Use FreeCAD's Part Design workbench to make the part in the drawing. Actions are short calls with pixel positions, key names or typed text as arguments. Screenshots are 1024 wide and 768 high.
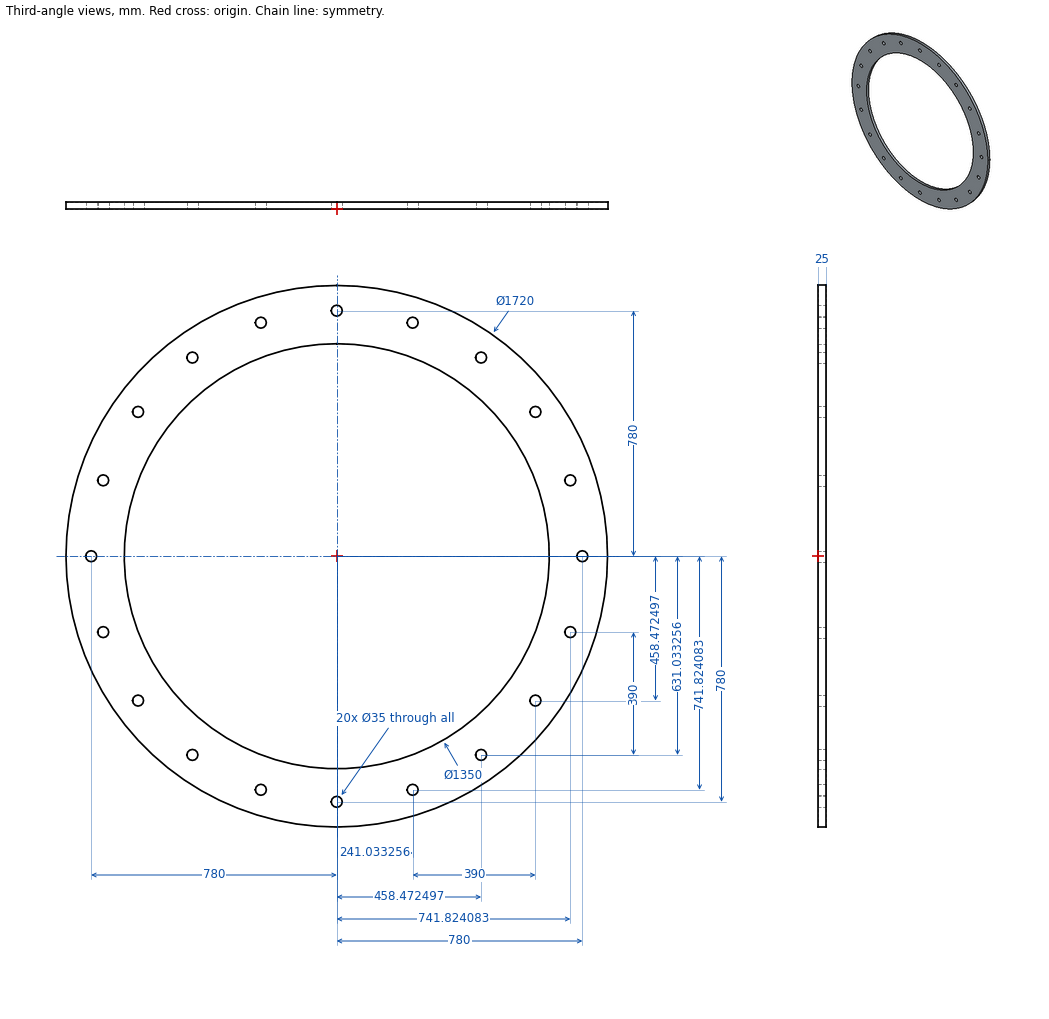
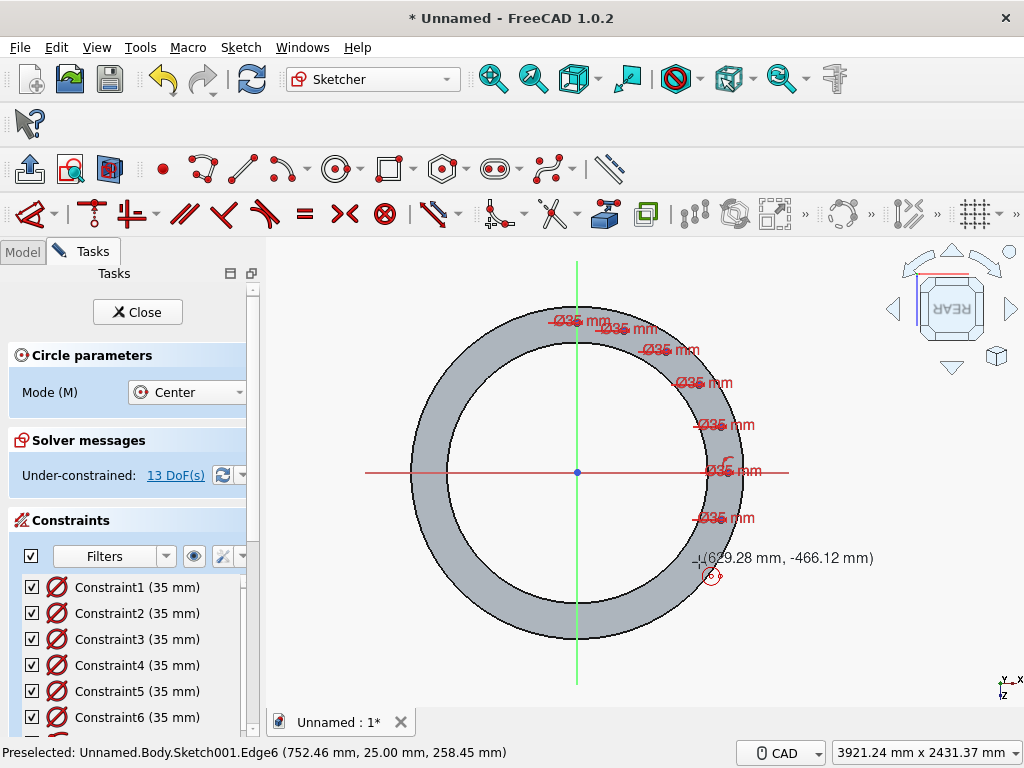
click(699, 562)
move(702, 559)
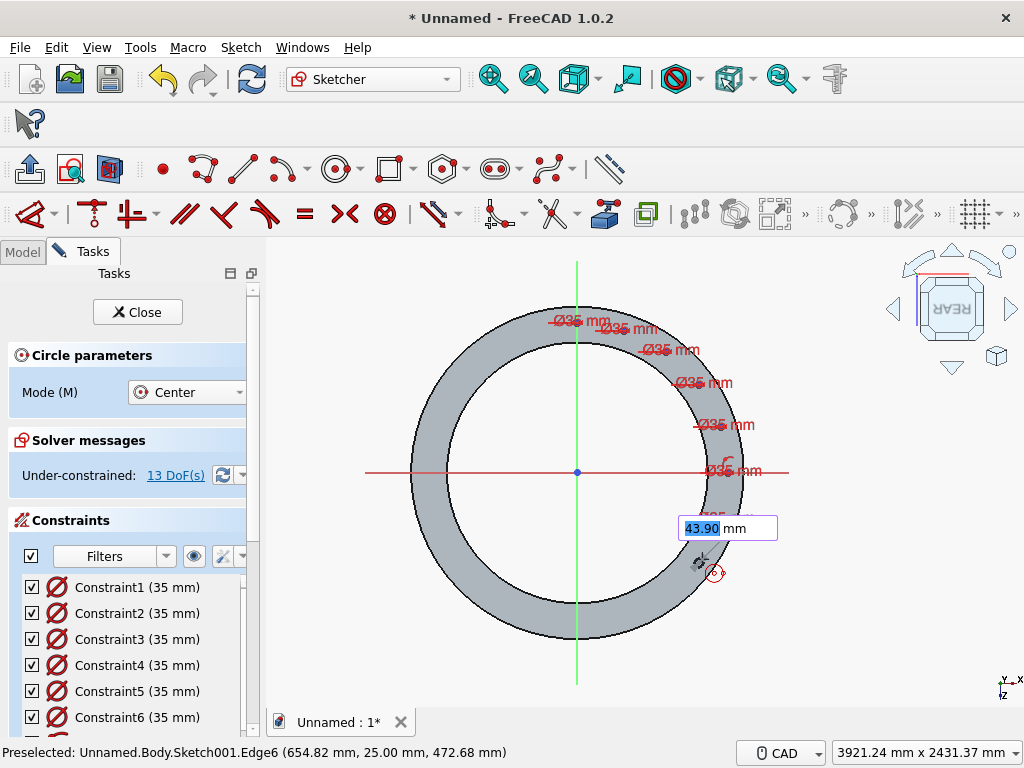
text(35)
key(Return)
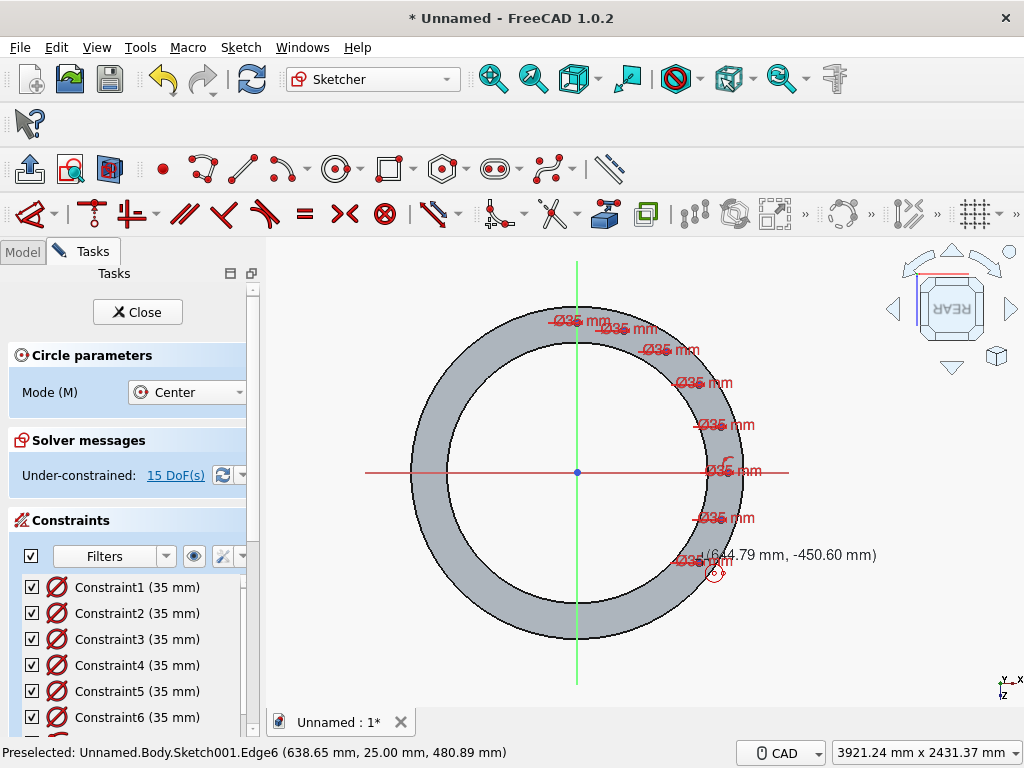
scroll(666, 595, up, 10)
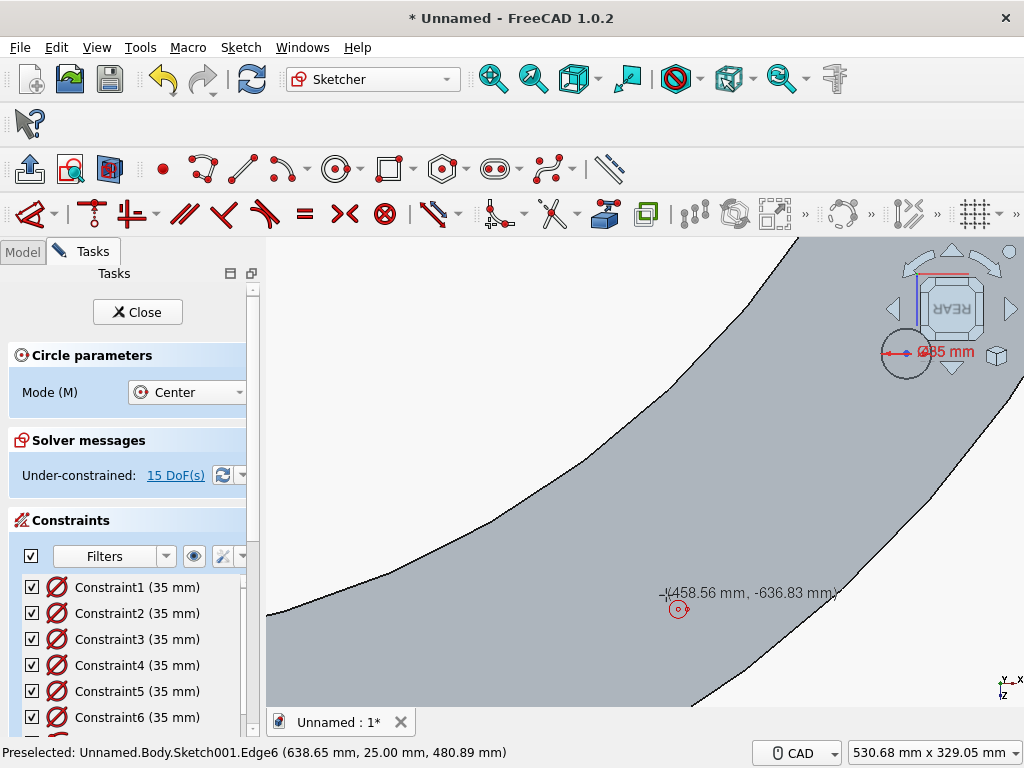
scroll(666, 595, down, 10)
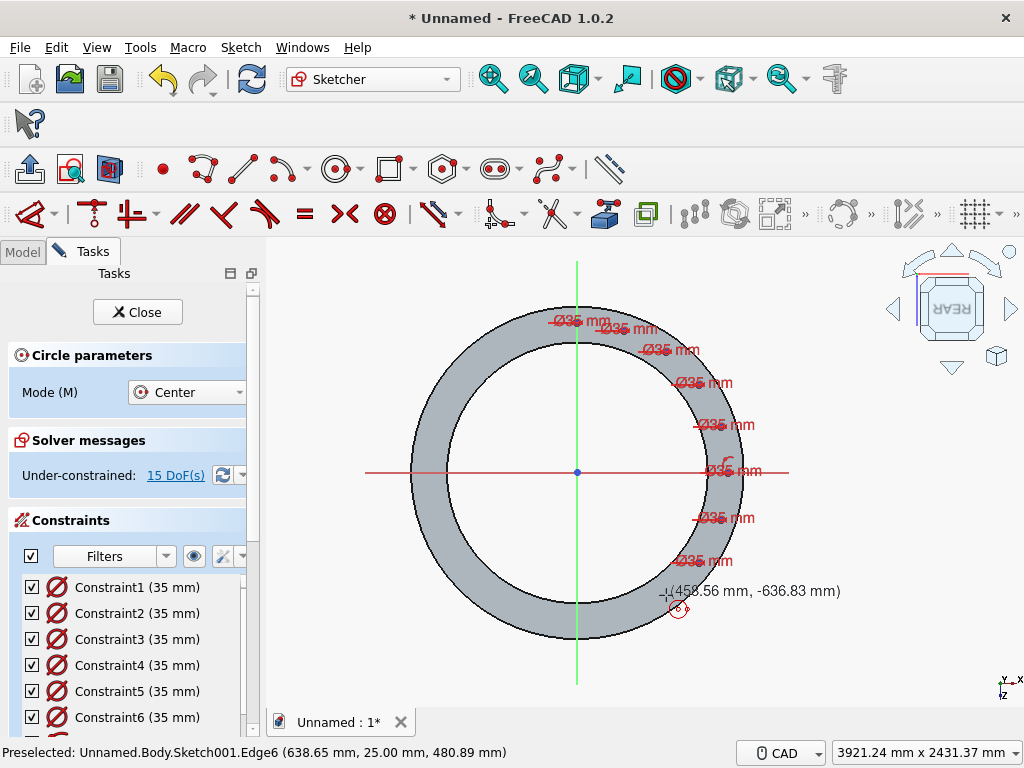
click(666, 595)
move(668, 592)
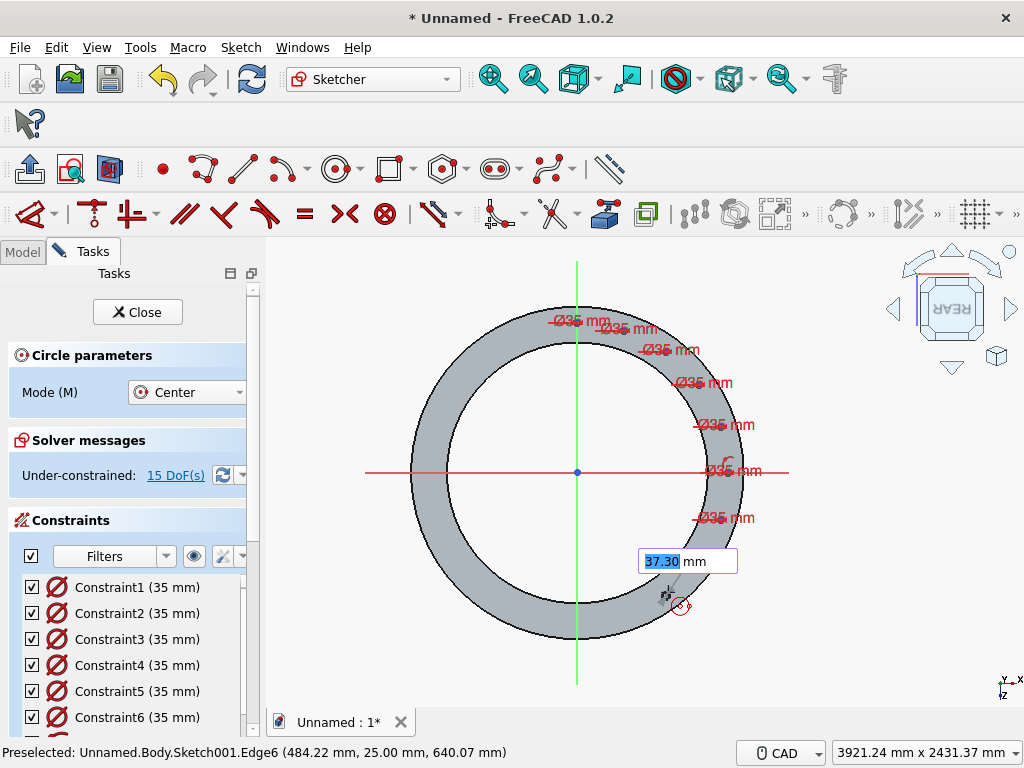
text(35)
key(Return)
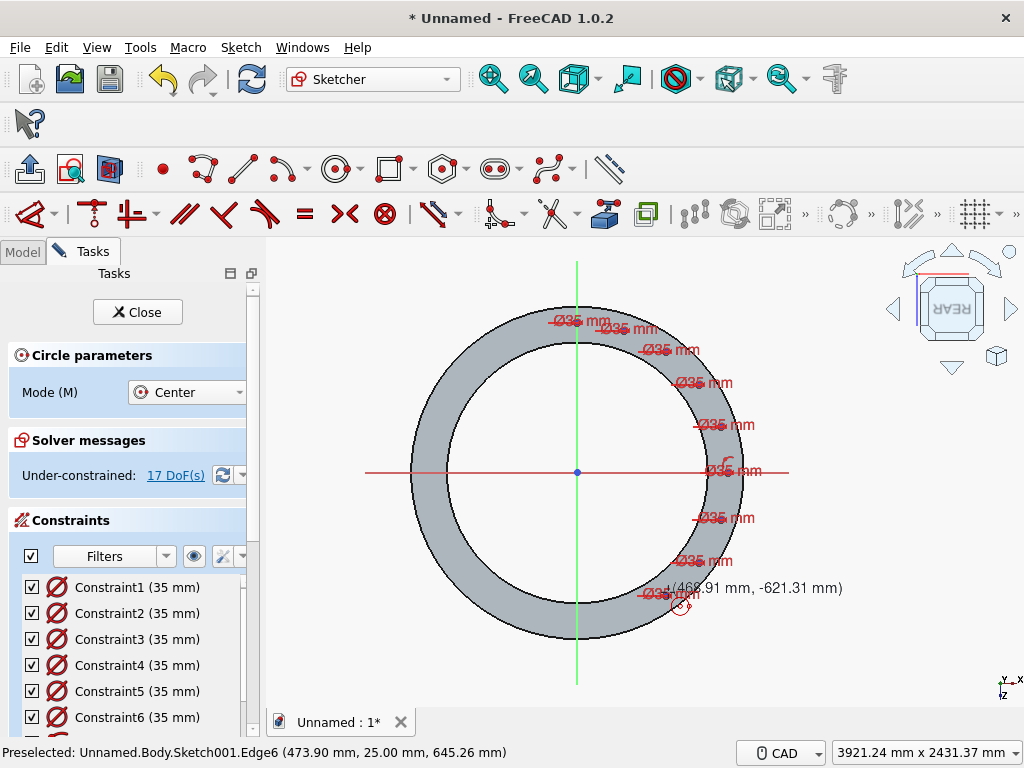
scroll(624, 616, up, 10)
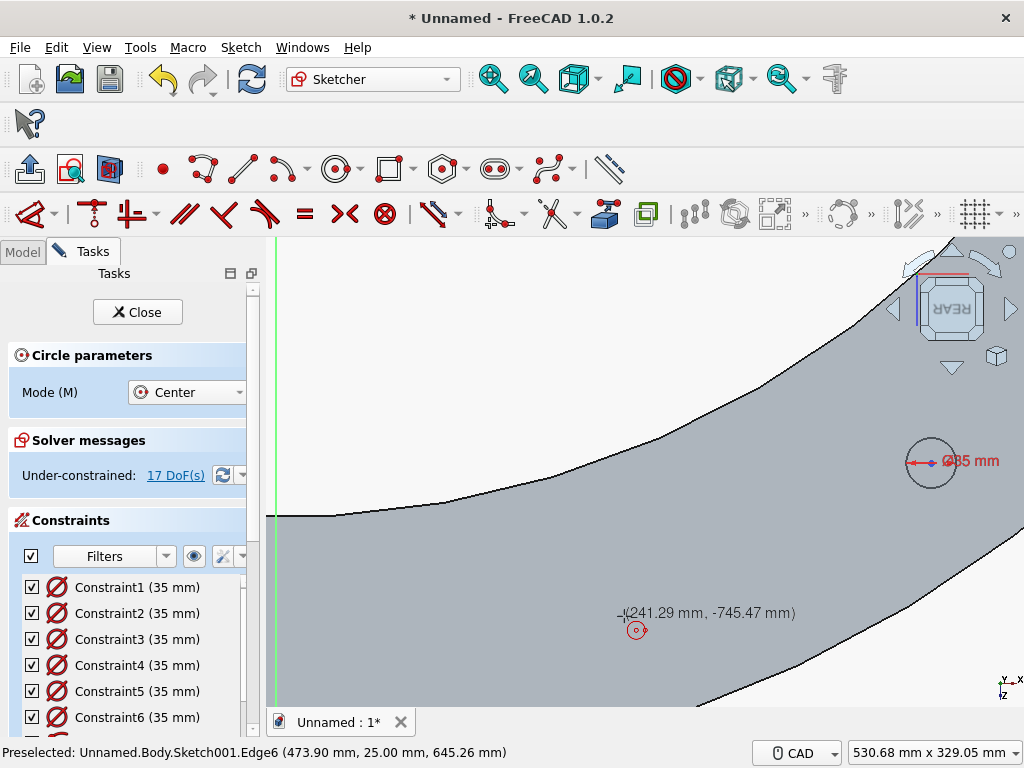
scroll(623, 616, down, 10)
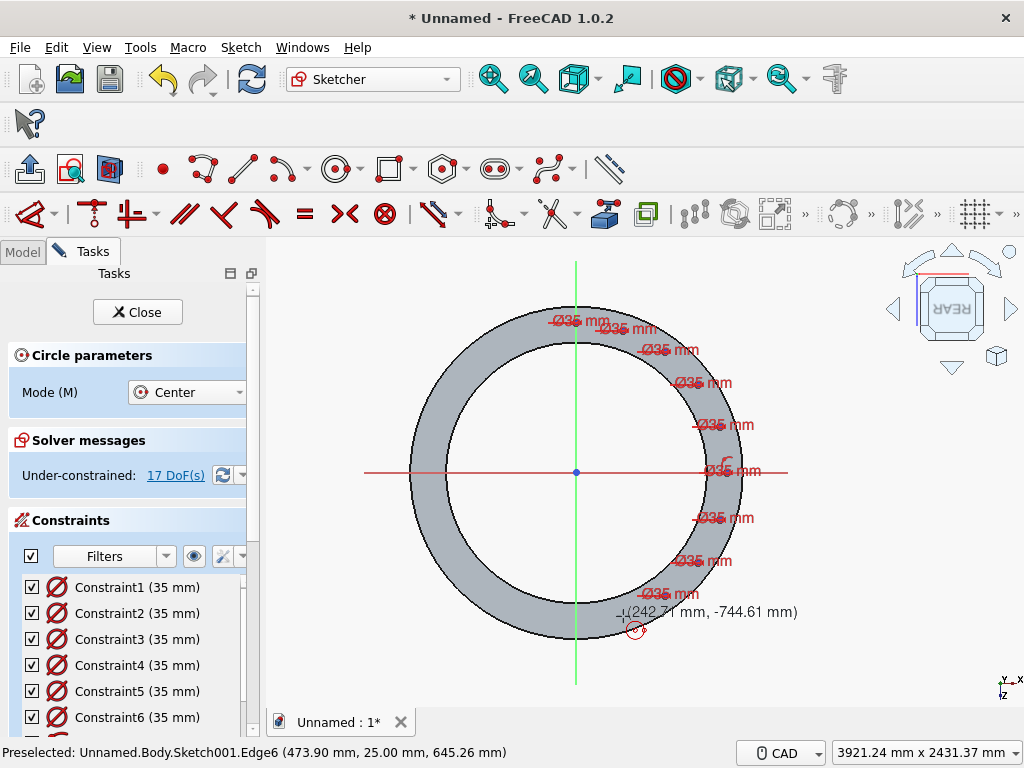
click(623, 616)
move(625, 614)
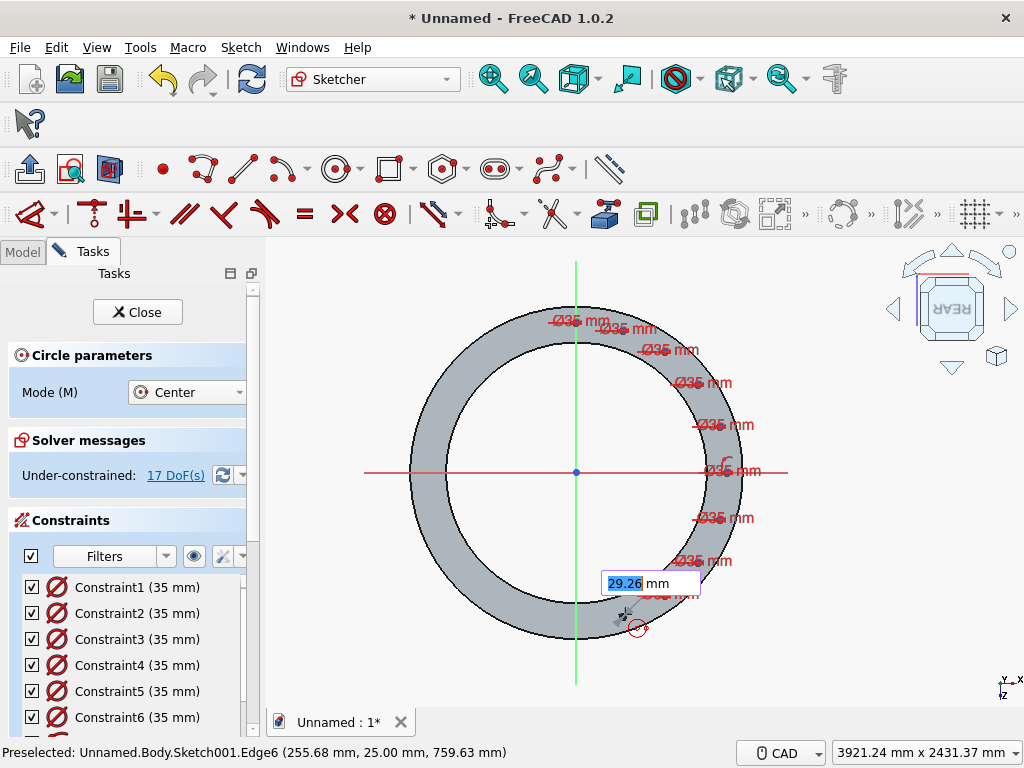
text(35)
key(Return)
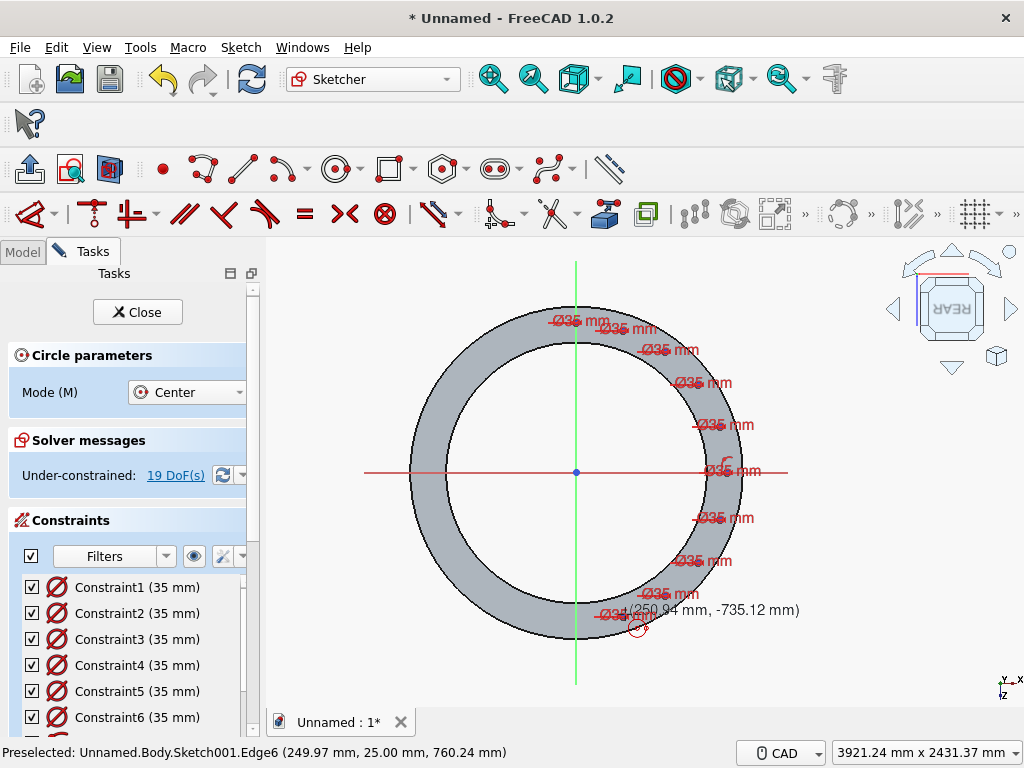
scroll(576, 624, up, 10)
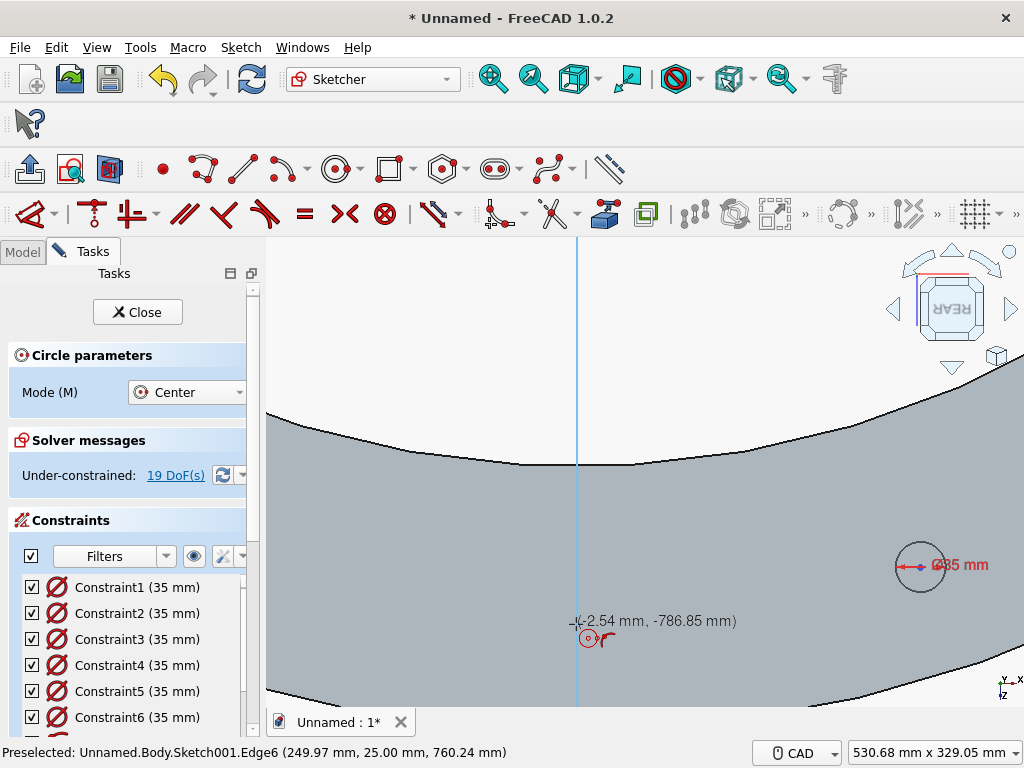
scroll(576, 624, down, 10)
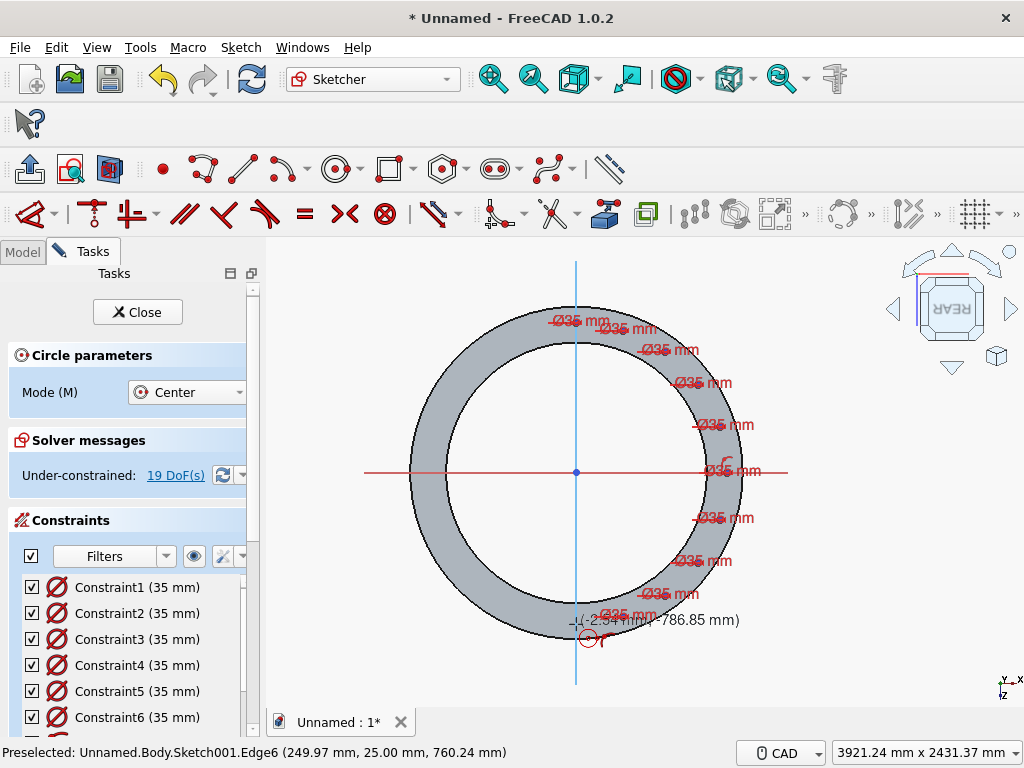
click(576, 624)